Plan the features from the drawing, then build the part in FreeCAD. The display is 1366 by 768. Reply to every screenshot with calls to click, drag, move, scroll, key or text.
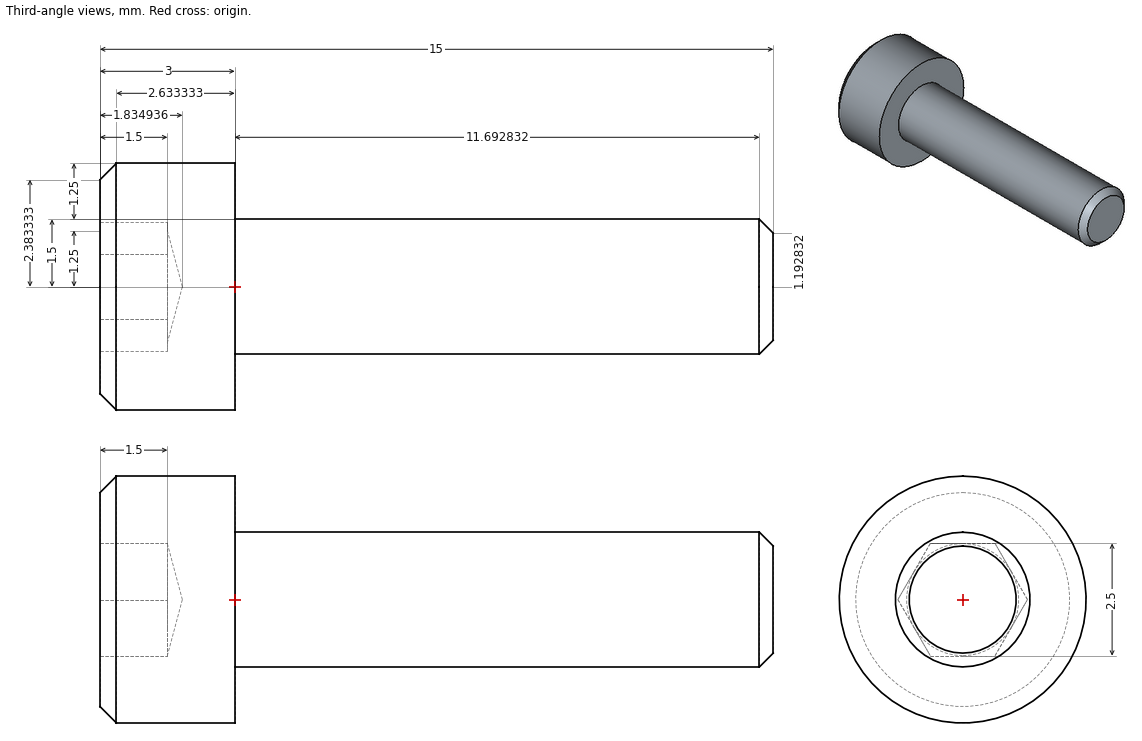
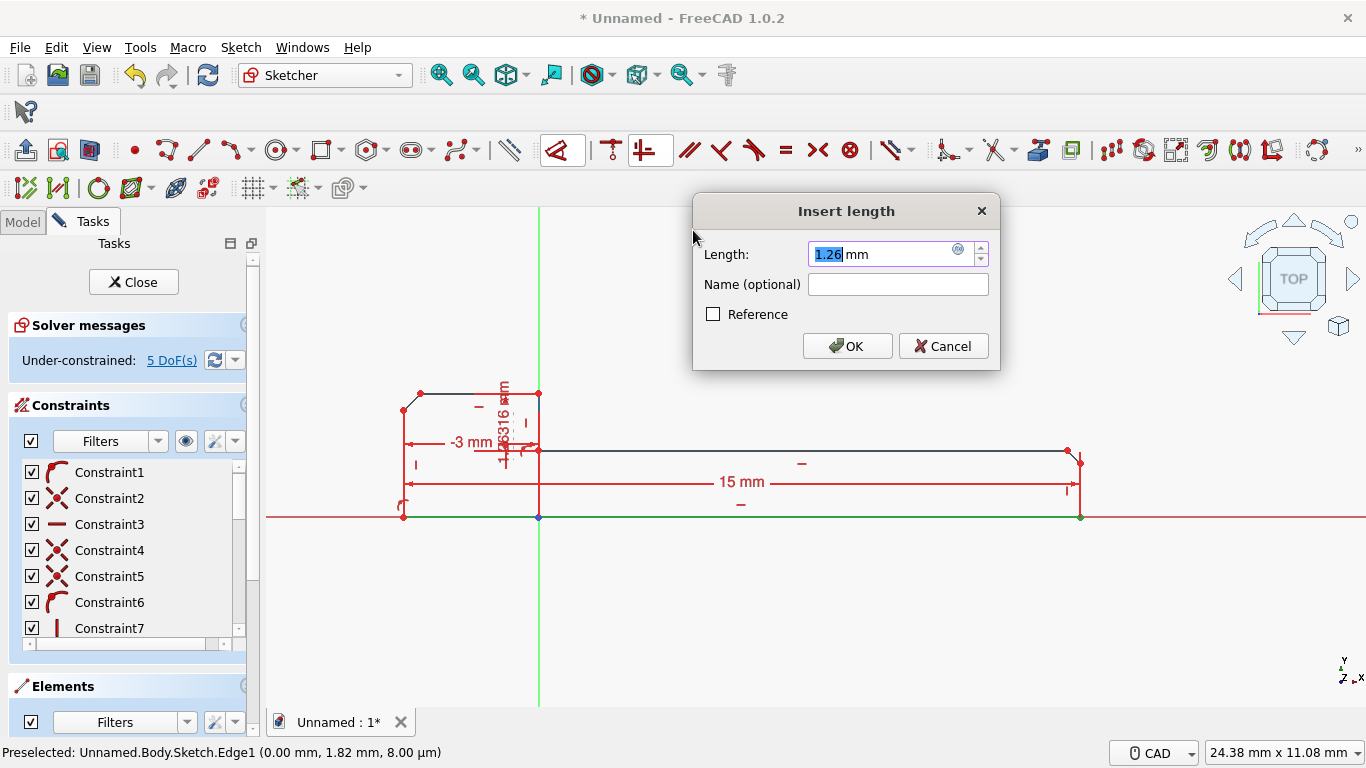
text(1.25)
key(Return)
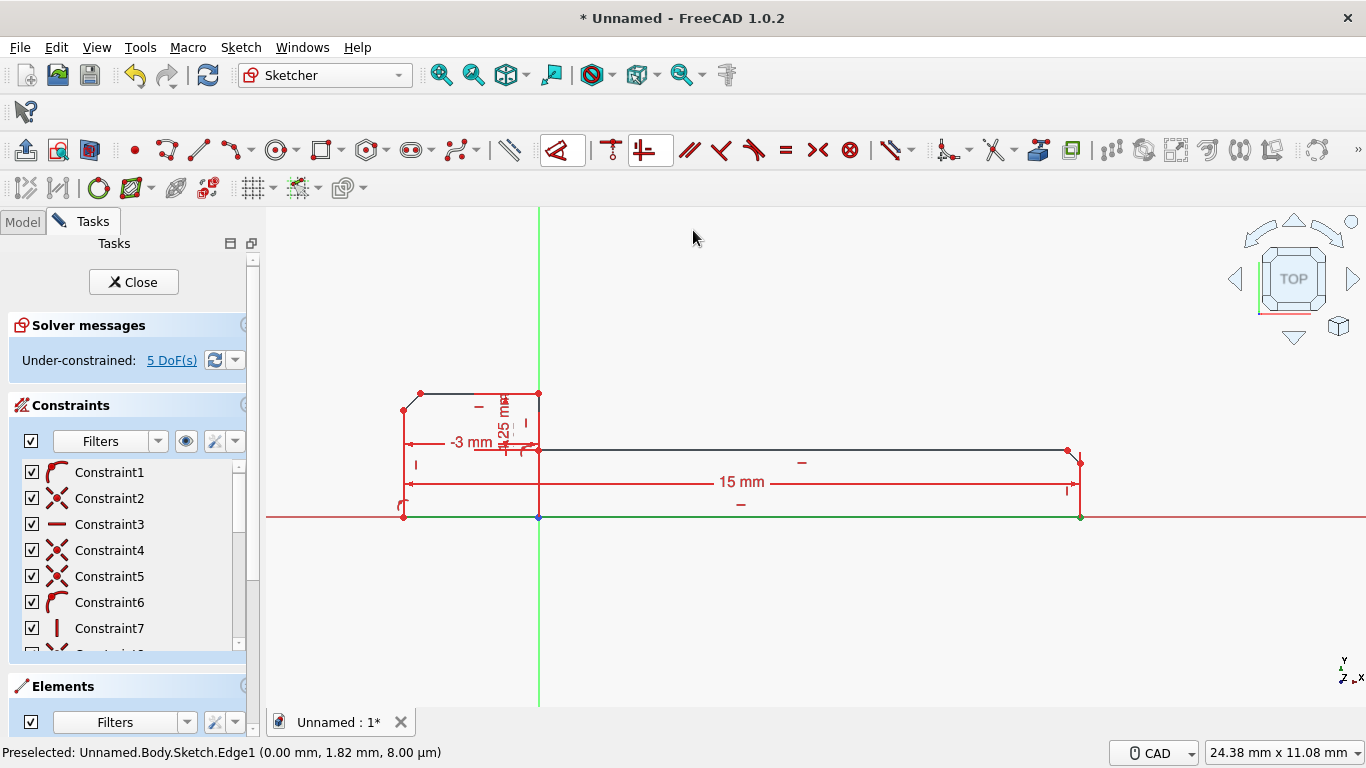
click(539, 450)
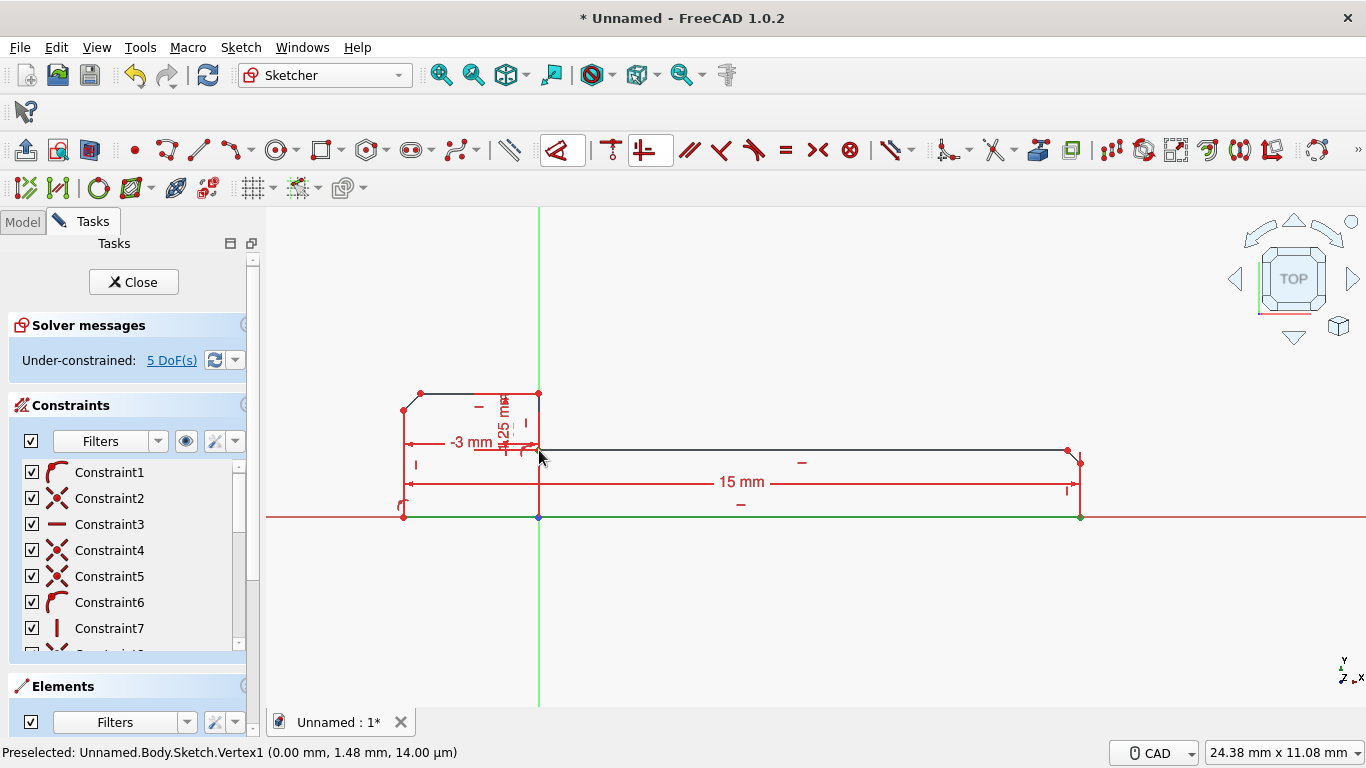
click(580, 150)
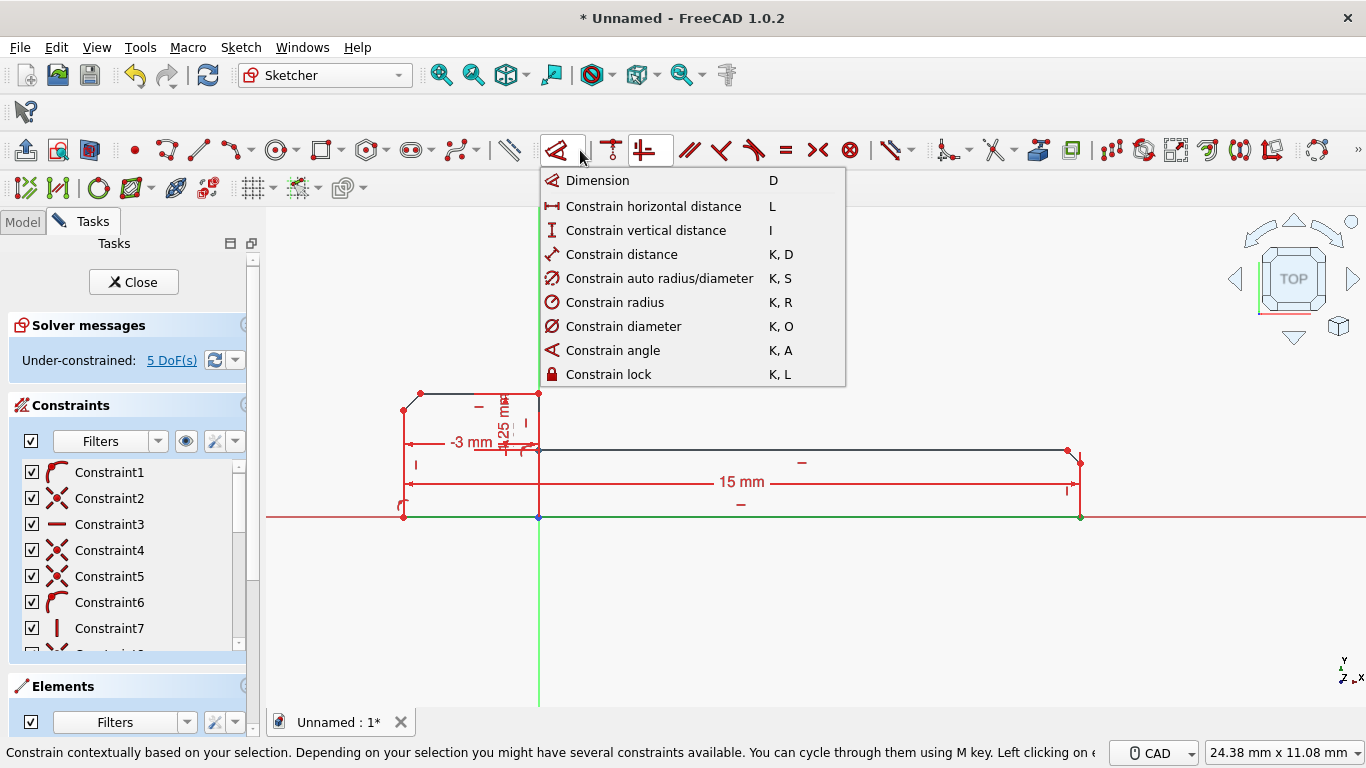
click(693, 230)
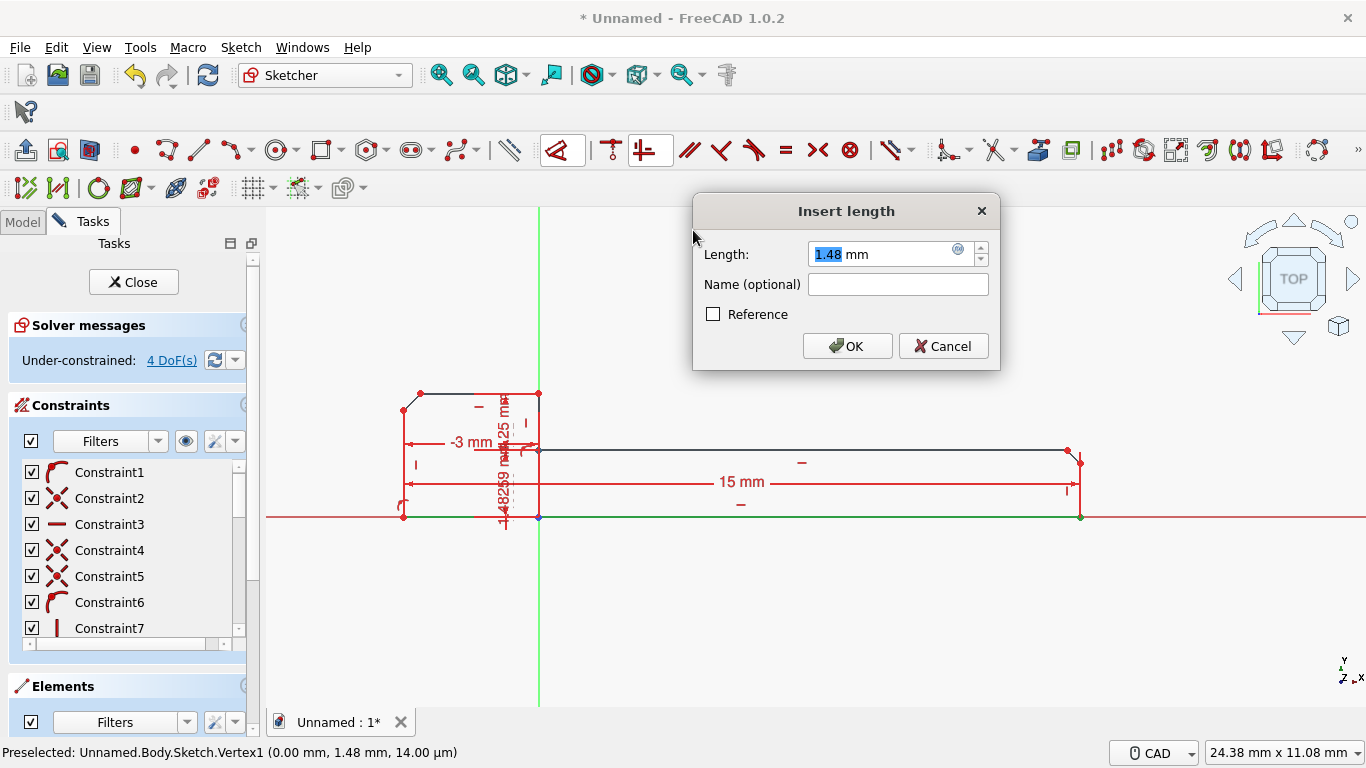
text(1.5)
key(Return)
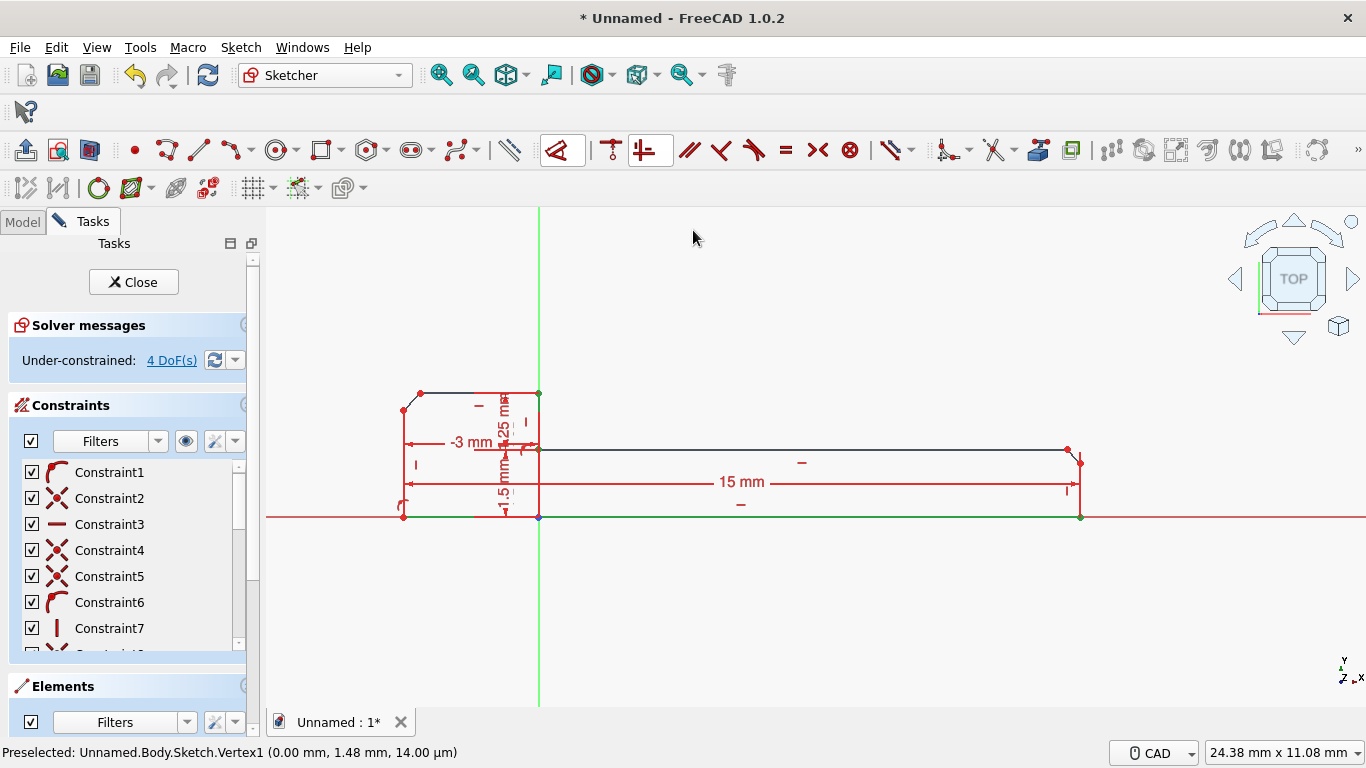
click(456, 393)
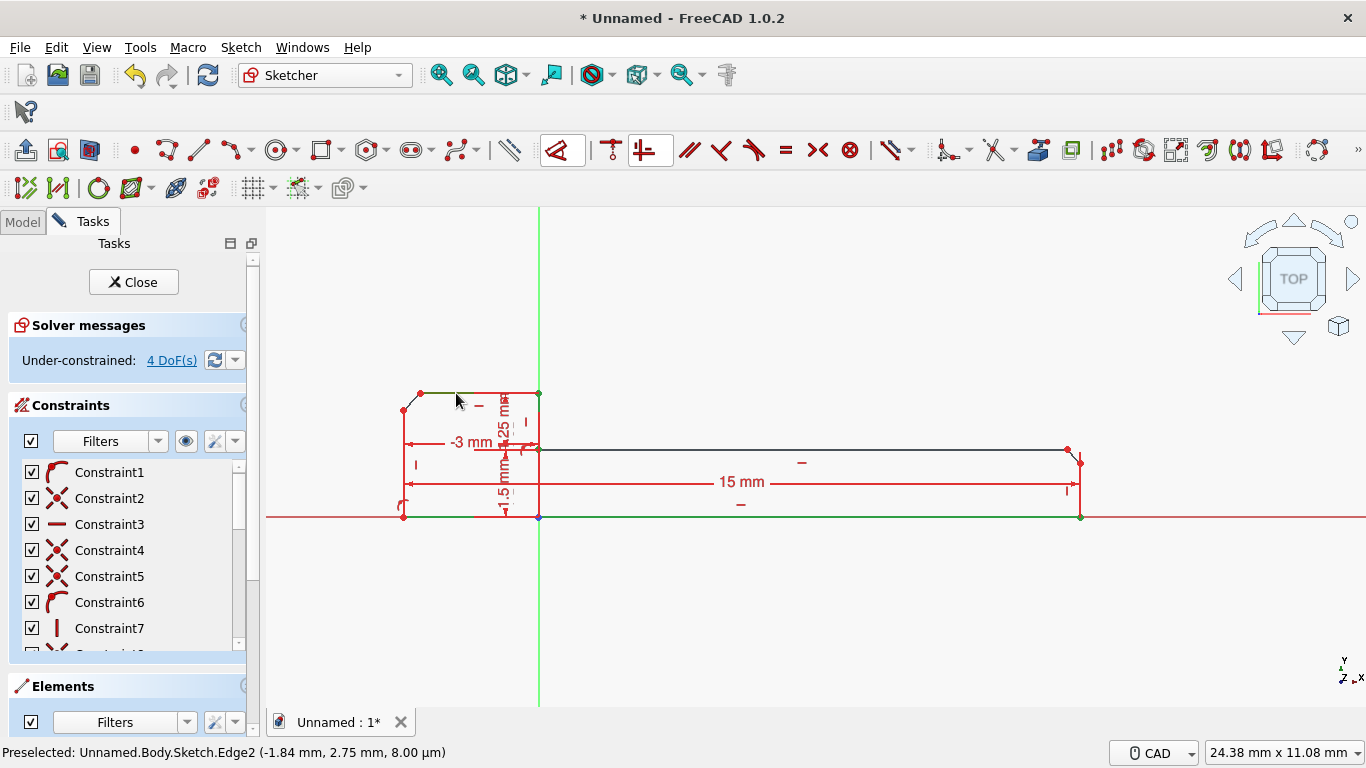
key(l)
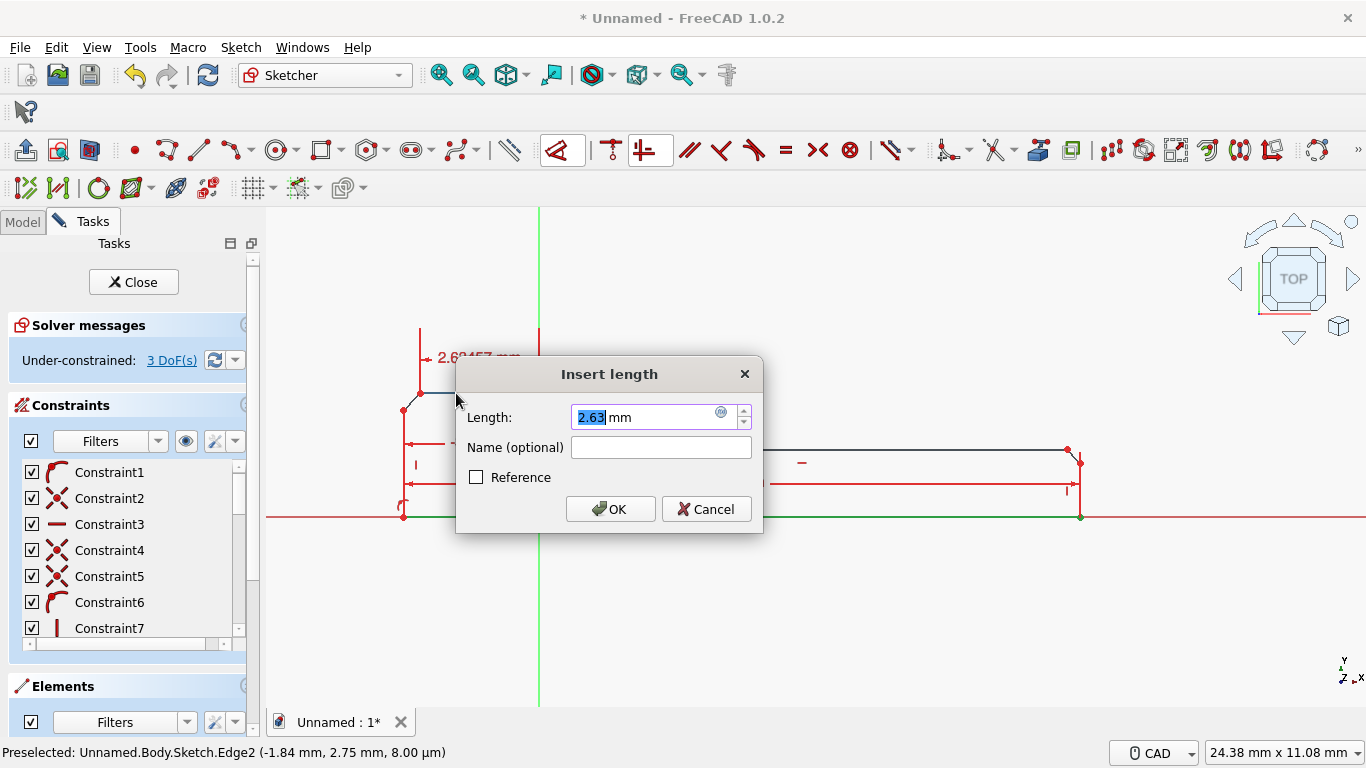
text(2.633333)
key(Return)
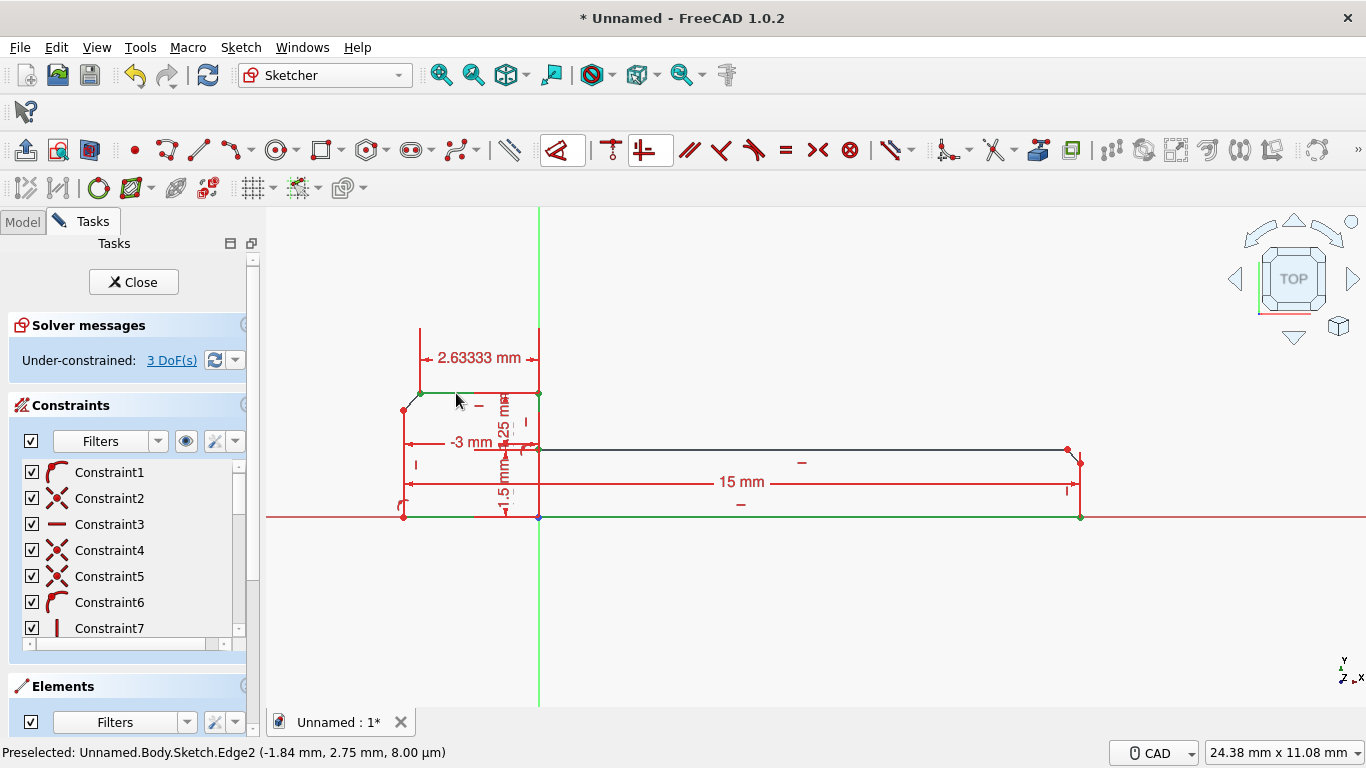
click(404, 443)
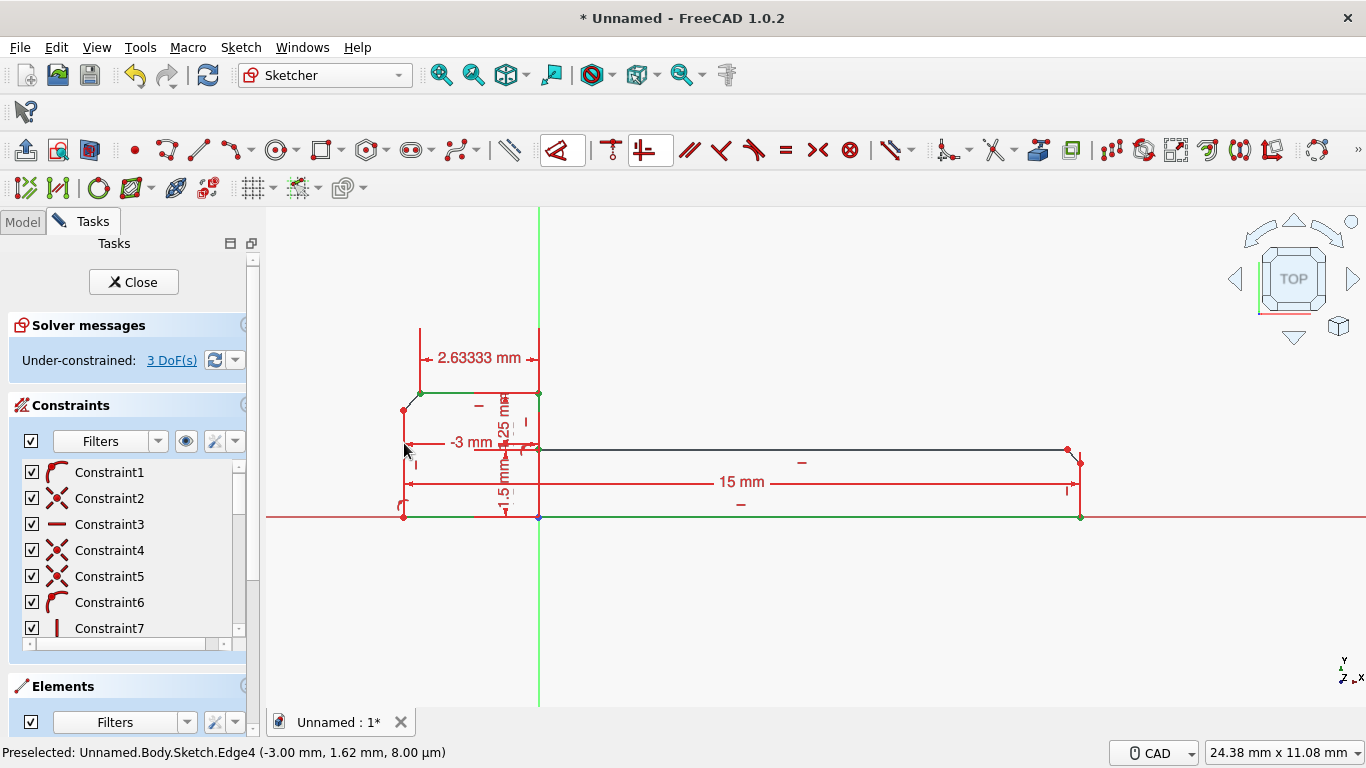
key(i)